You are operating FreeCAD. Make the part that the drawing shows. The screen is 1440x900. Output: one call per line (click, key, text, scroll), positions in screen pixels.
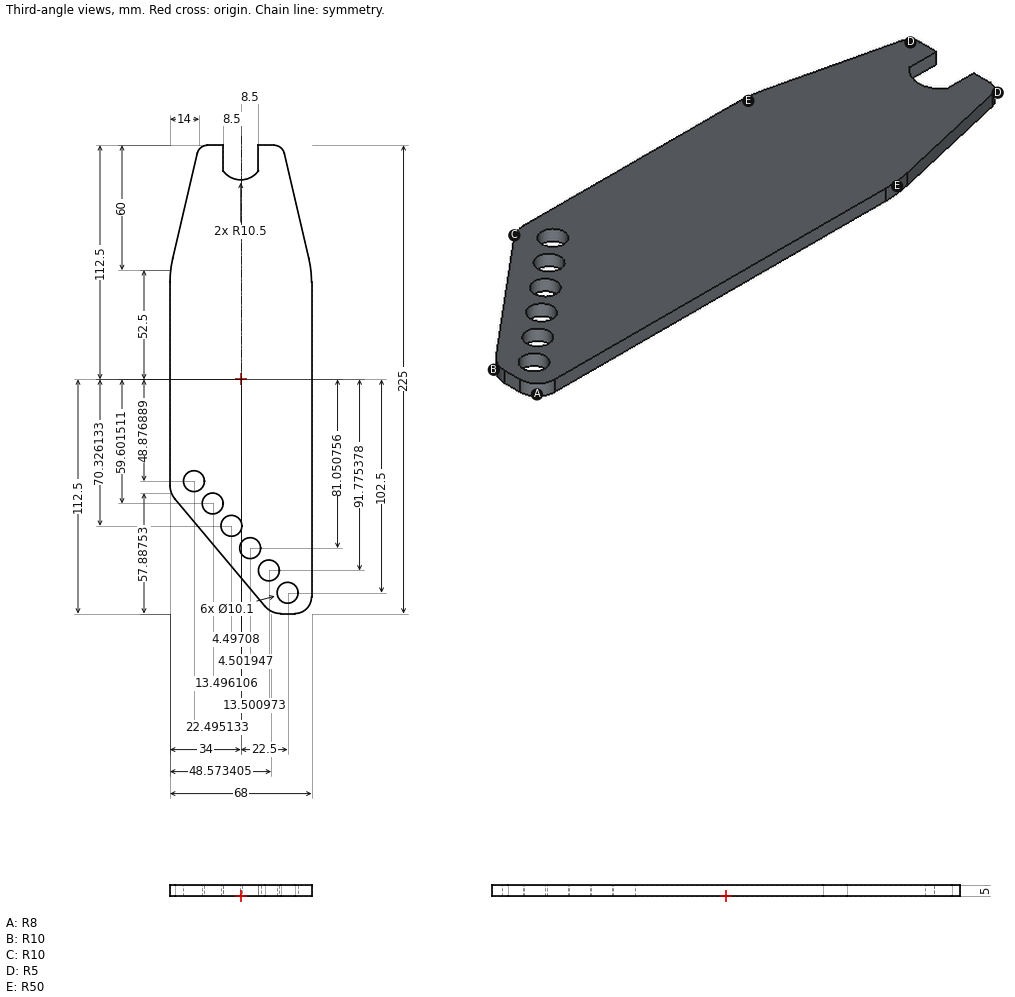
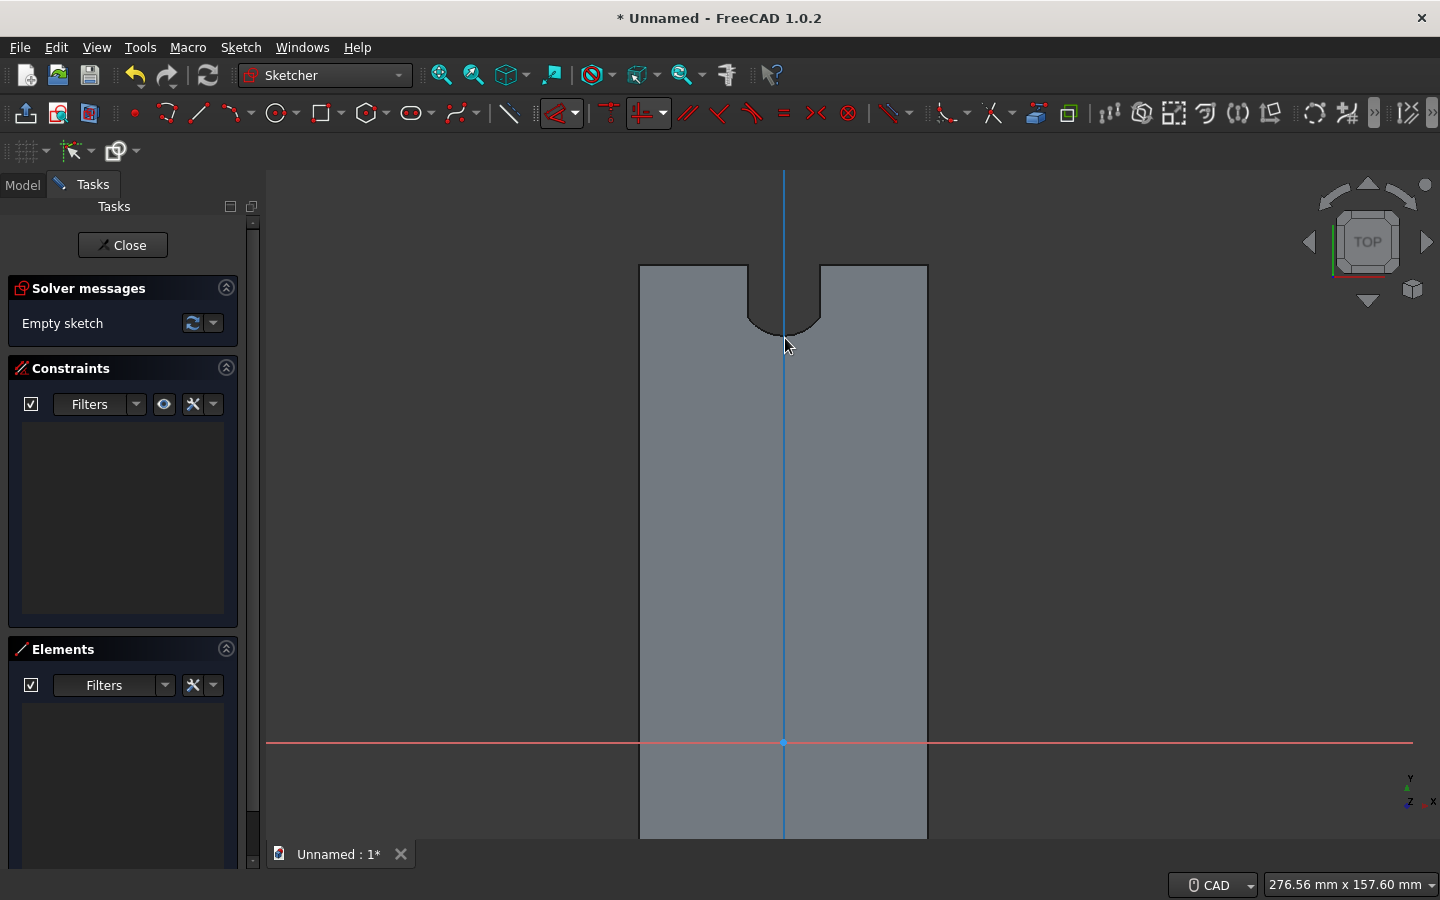
key(g)
key(m)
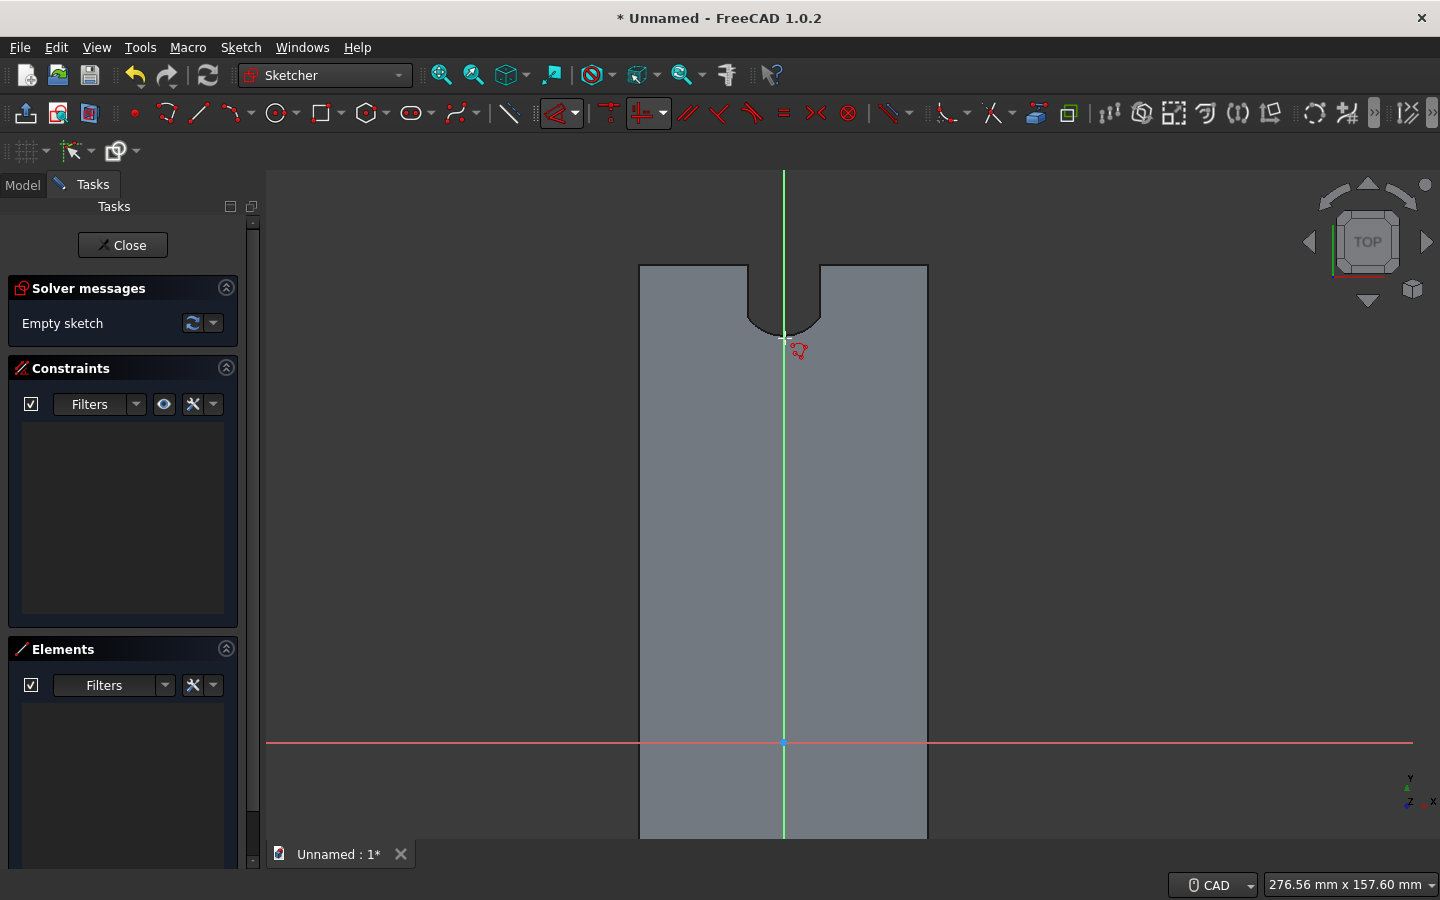
click(639, 520)
click(699, 265)
click(639, 265)
click(639, 521)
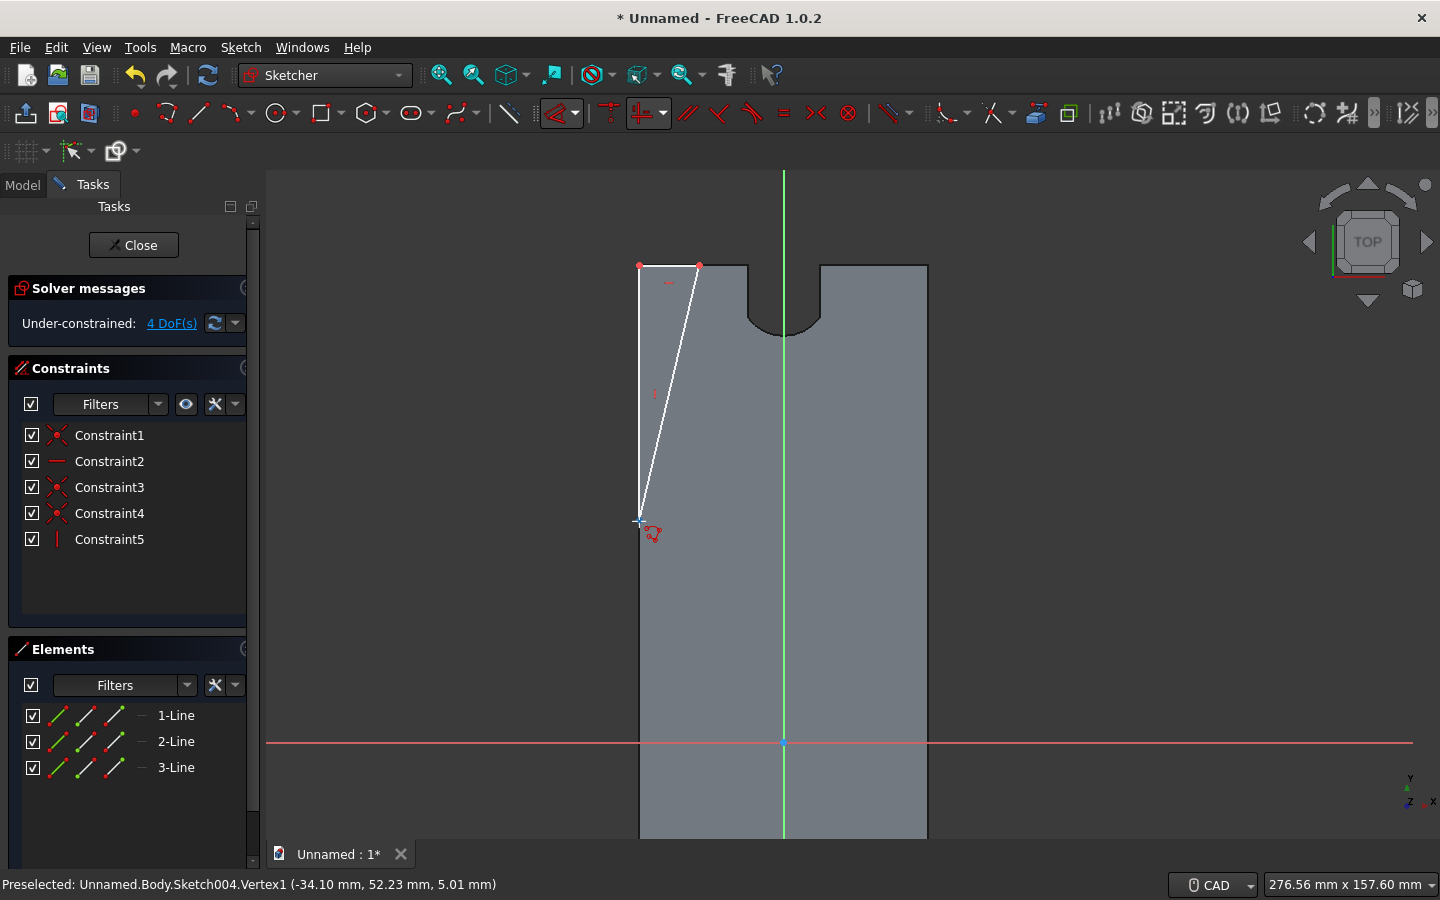
click(928, 520)
click(928, 265)
click(869, 265)
click(928, 521)
key(Escape)
key(Escape)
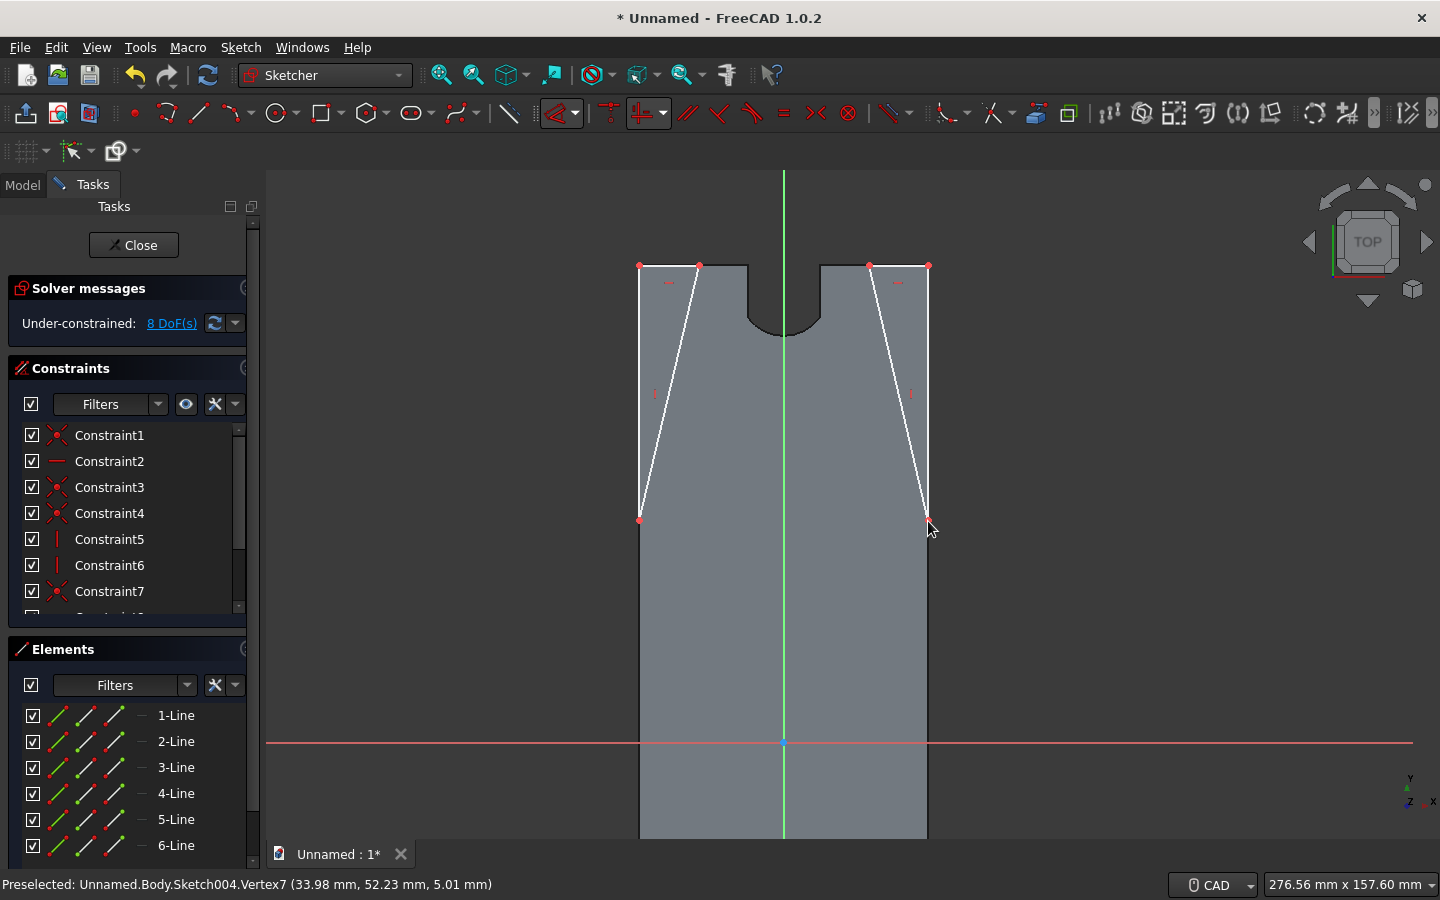
click(639, 521)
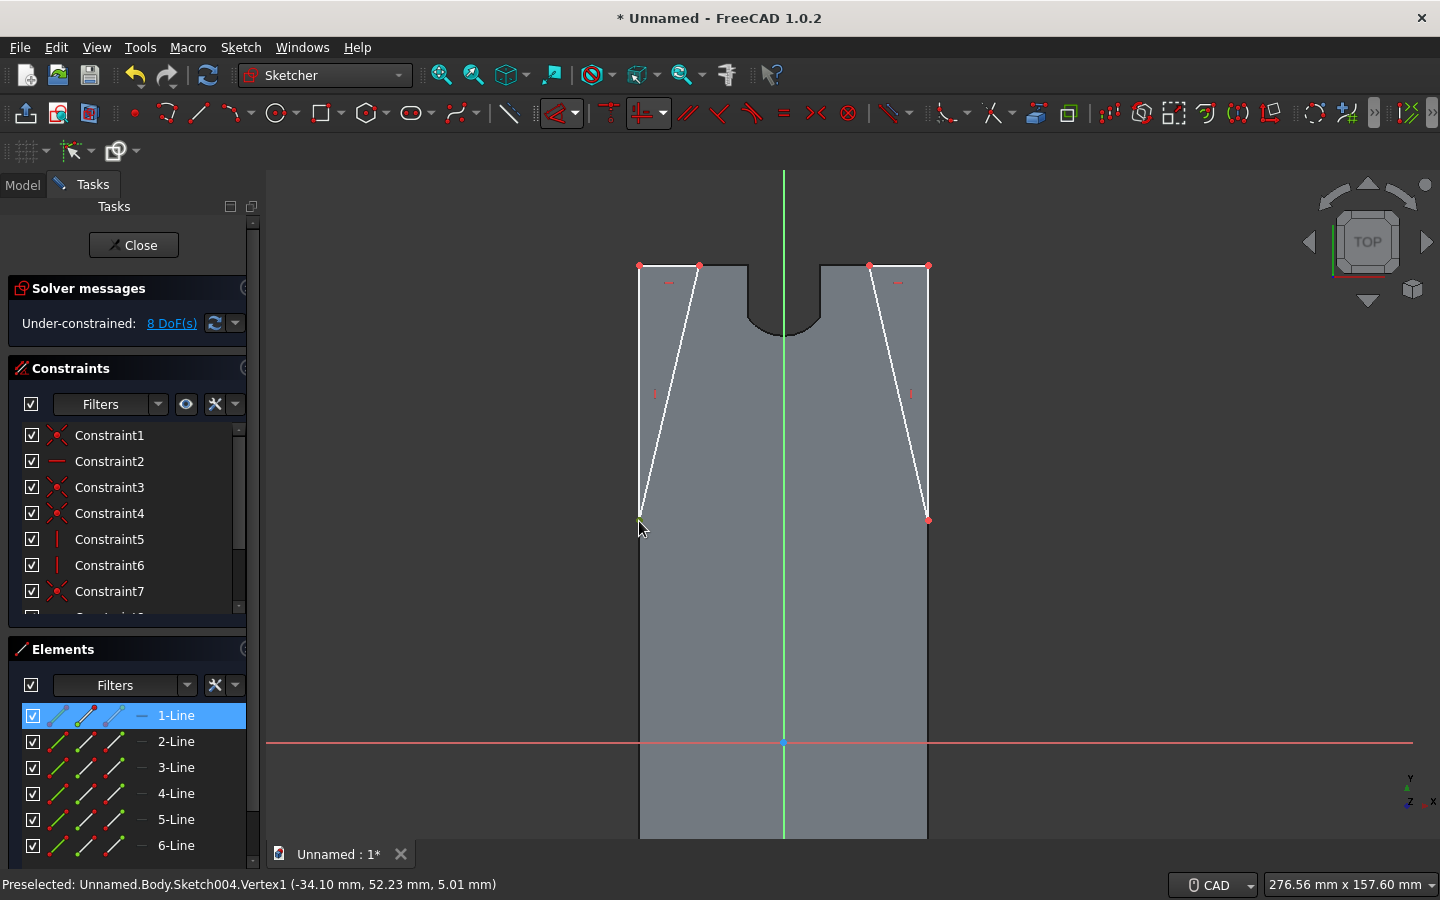
click(928, 521)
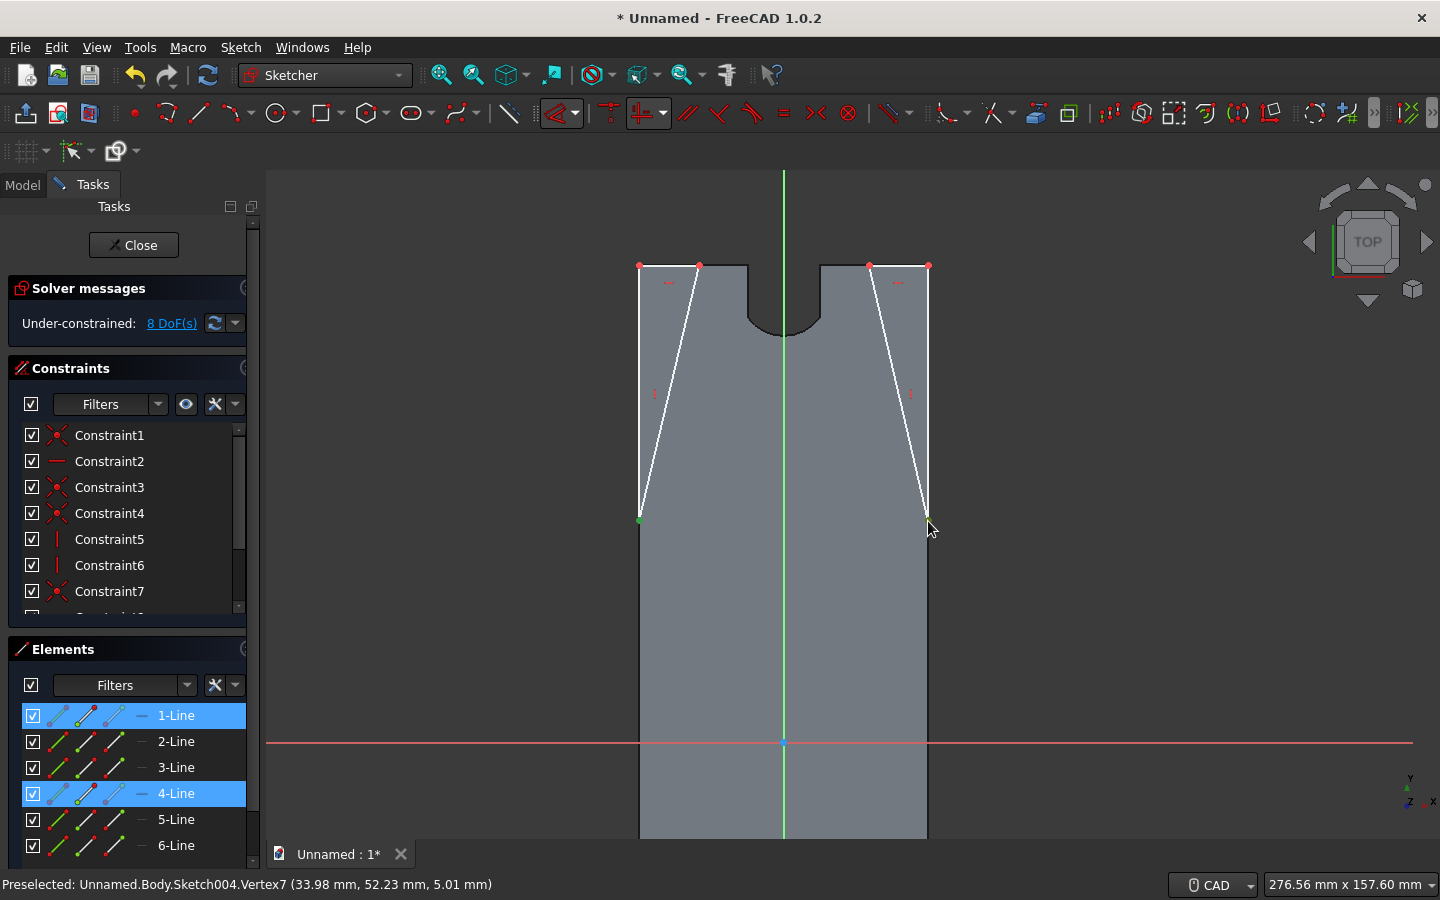
click(784, 680)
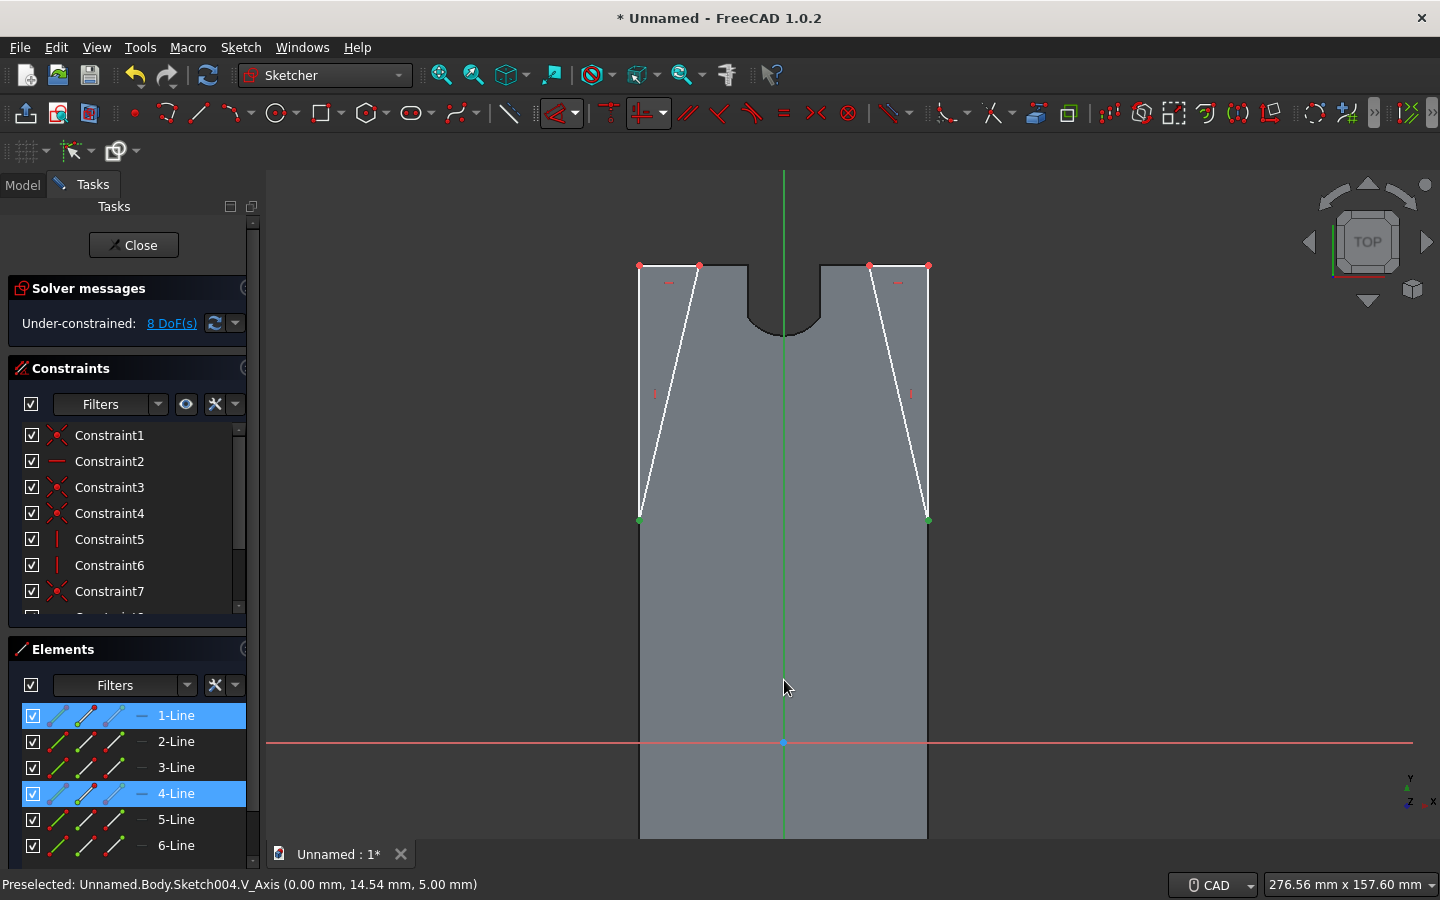
key(s)